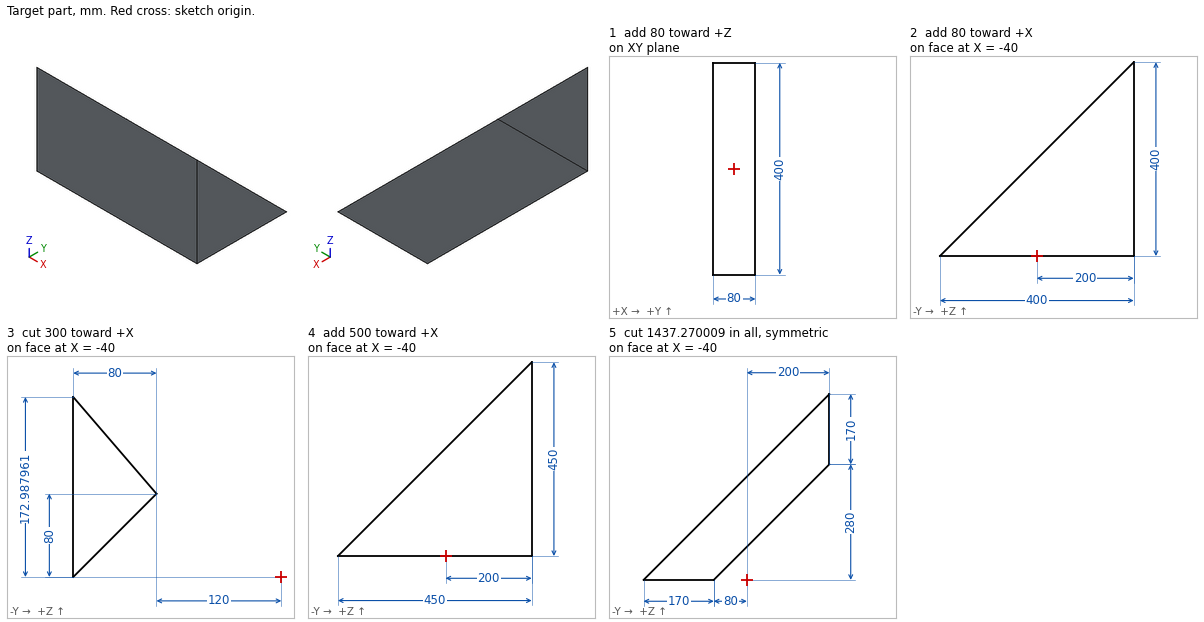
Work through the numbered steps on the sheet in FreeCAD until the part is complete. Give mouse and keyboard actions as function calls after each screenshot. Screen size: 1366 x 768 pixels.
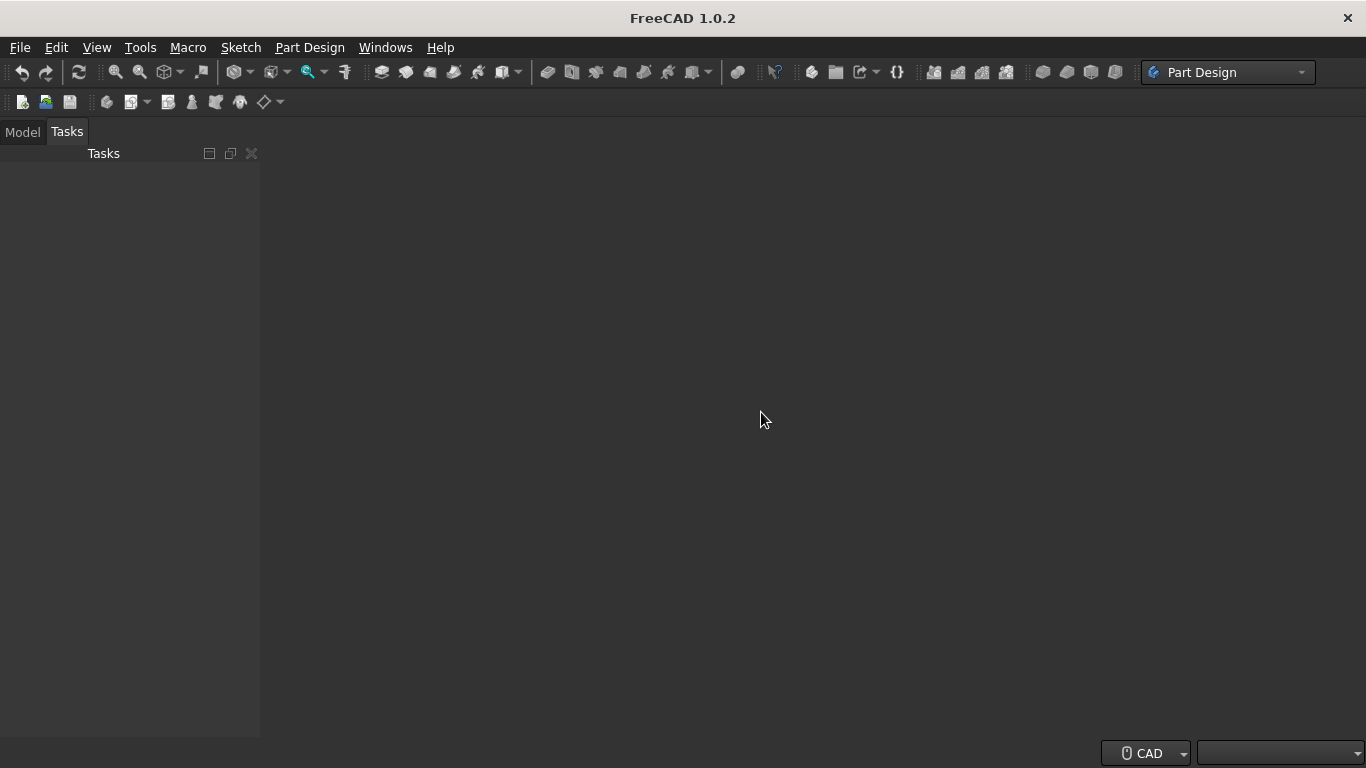
click(22, 102)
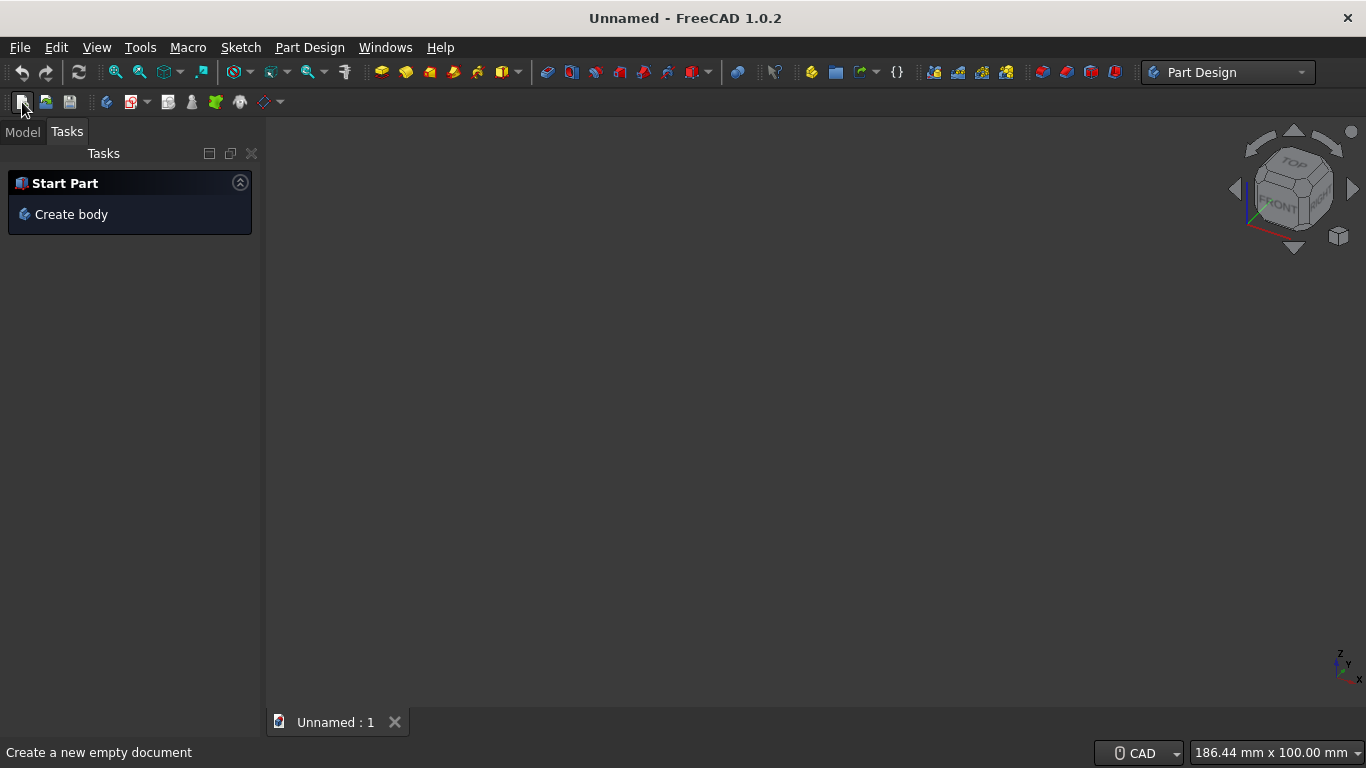
click(132, 102)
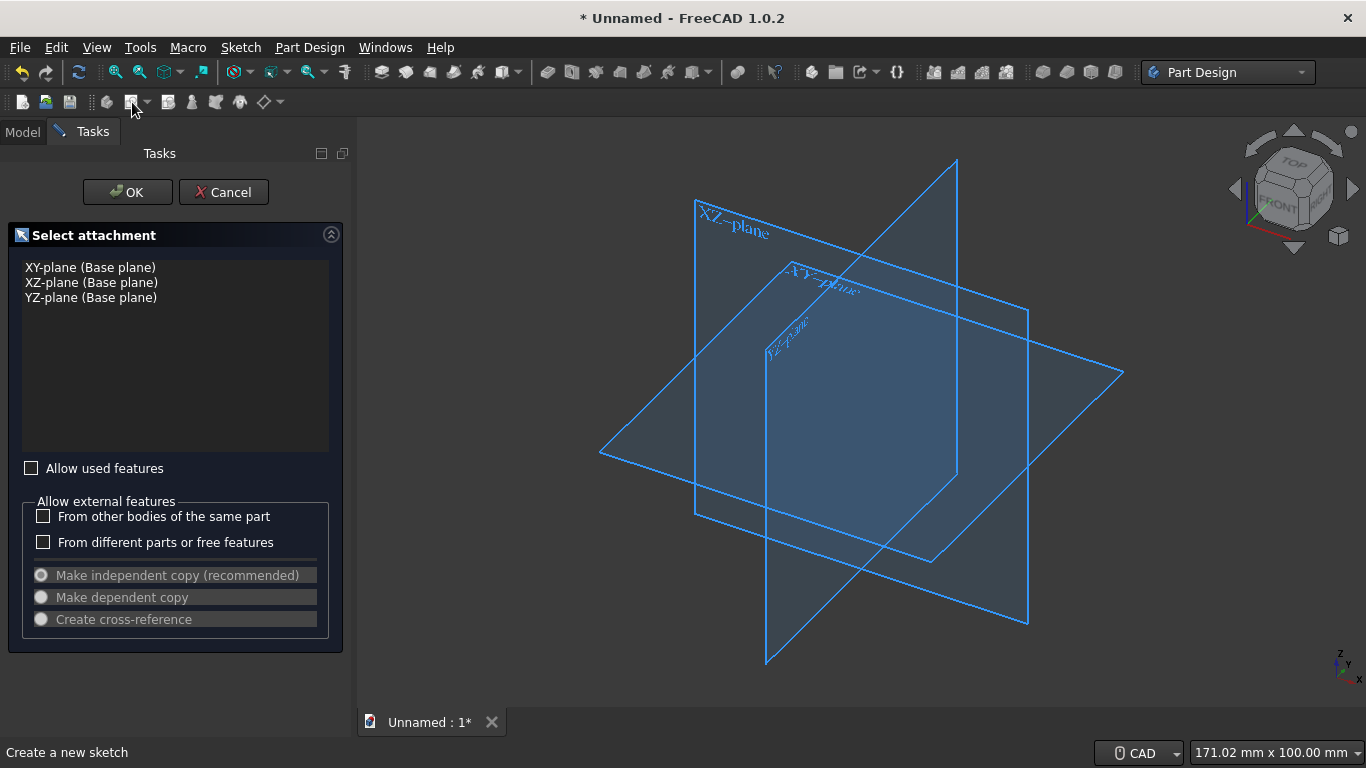
click(82, 268)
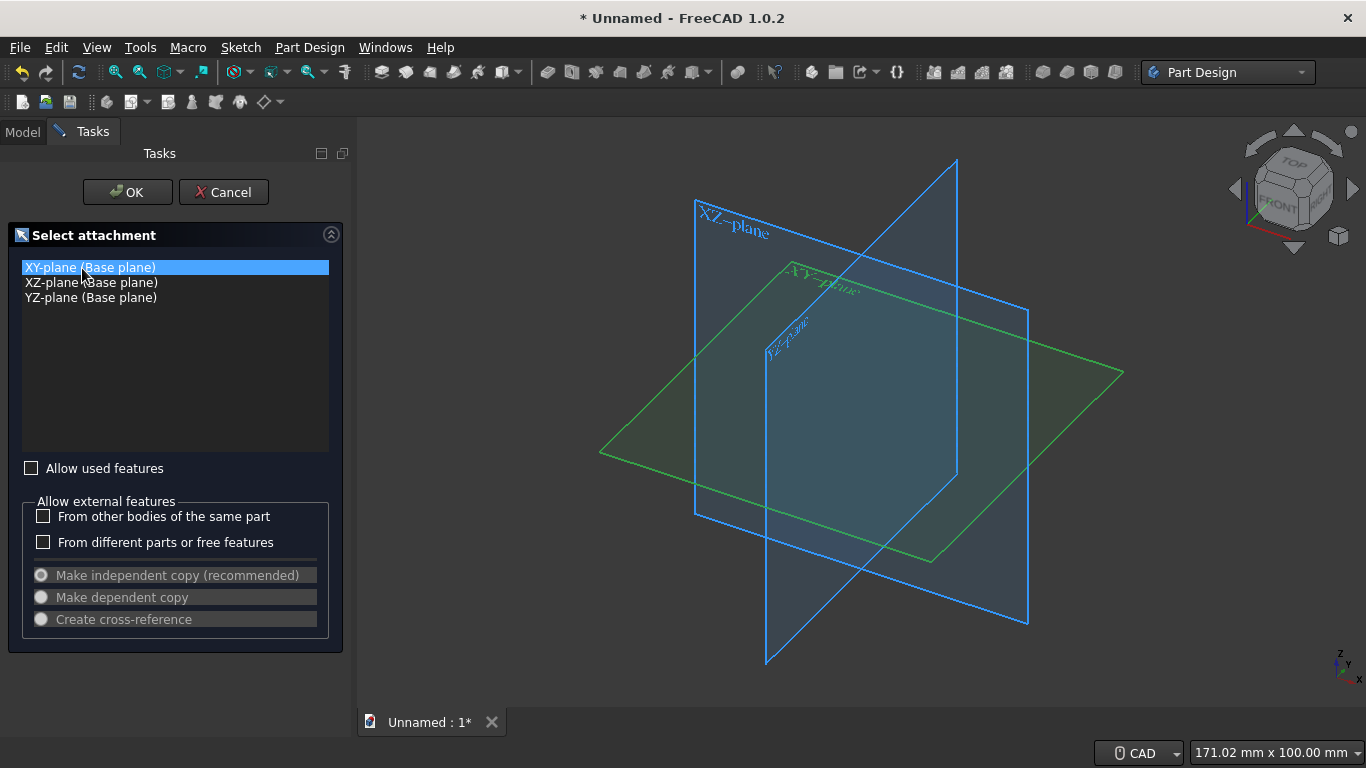
click(128, 192)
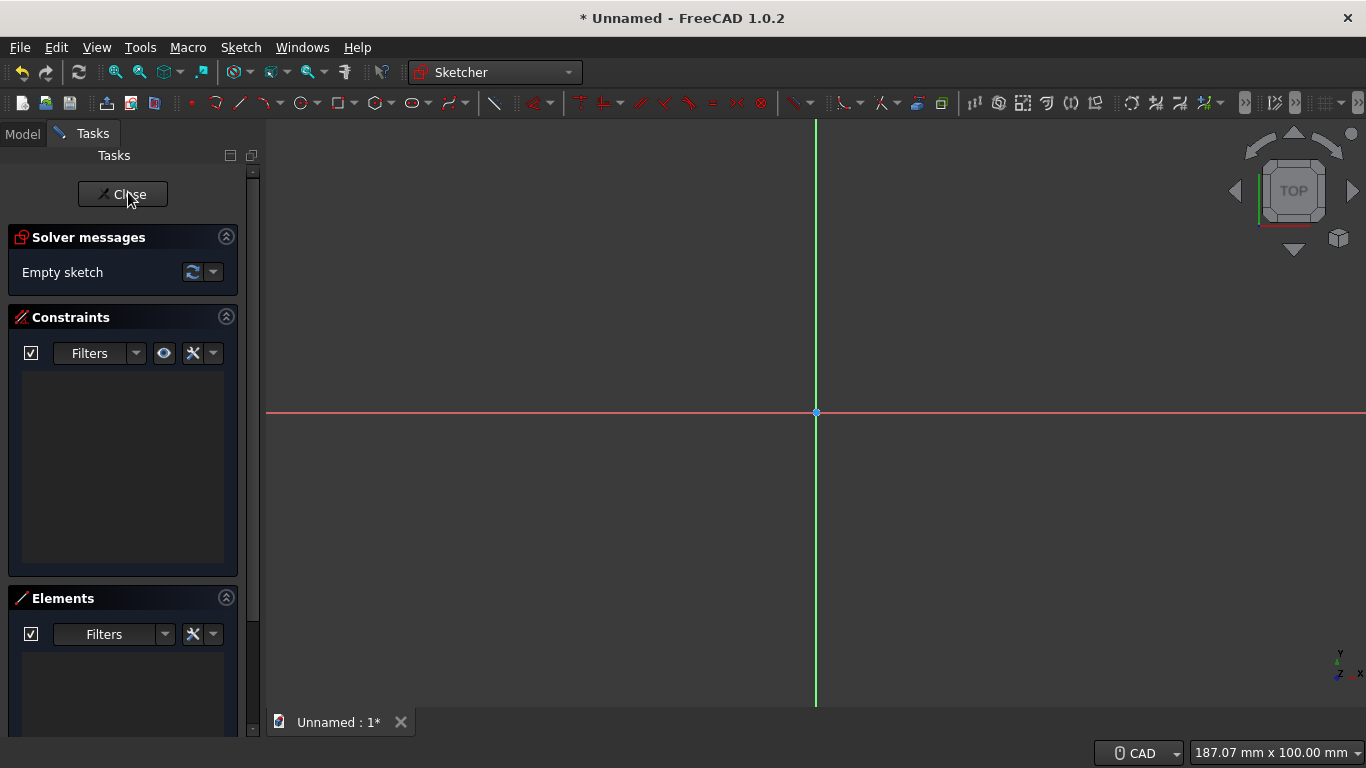
scroll(734, 413, down, 9)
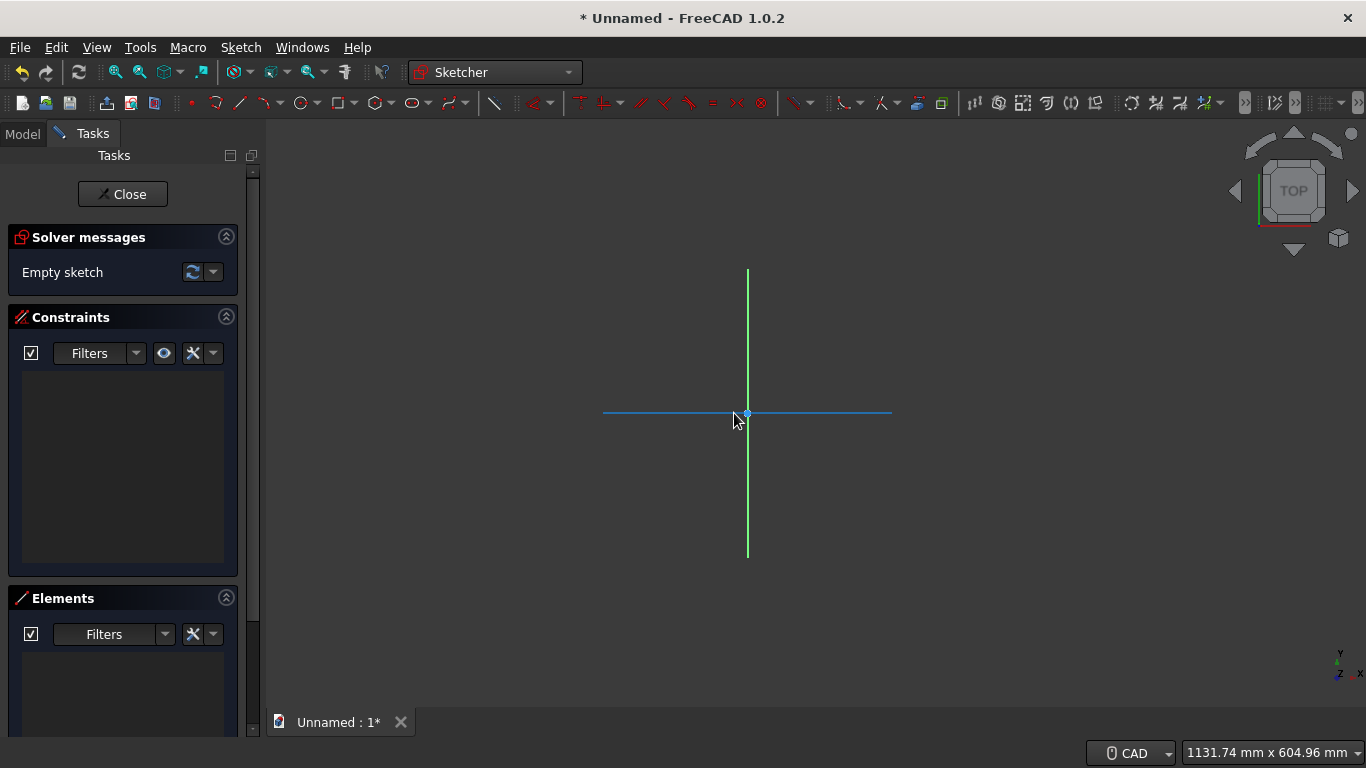
click(356, 104)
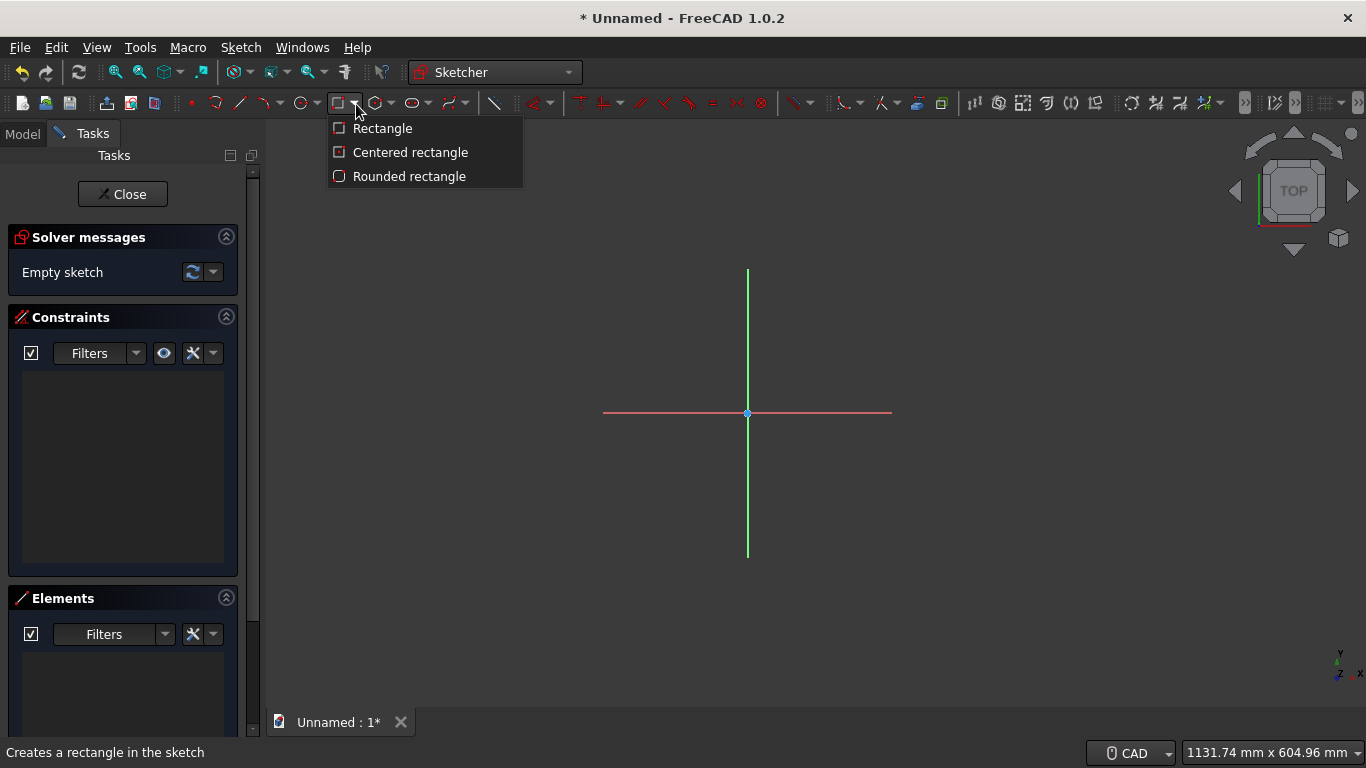
click(426, 152)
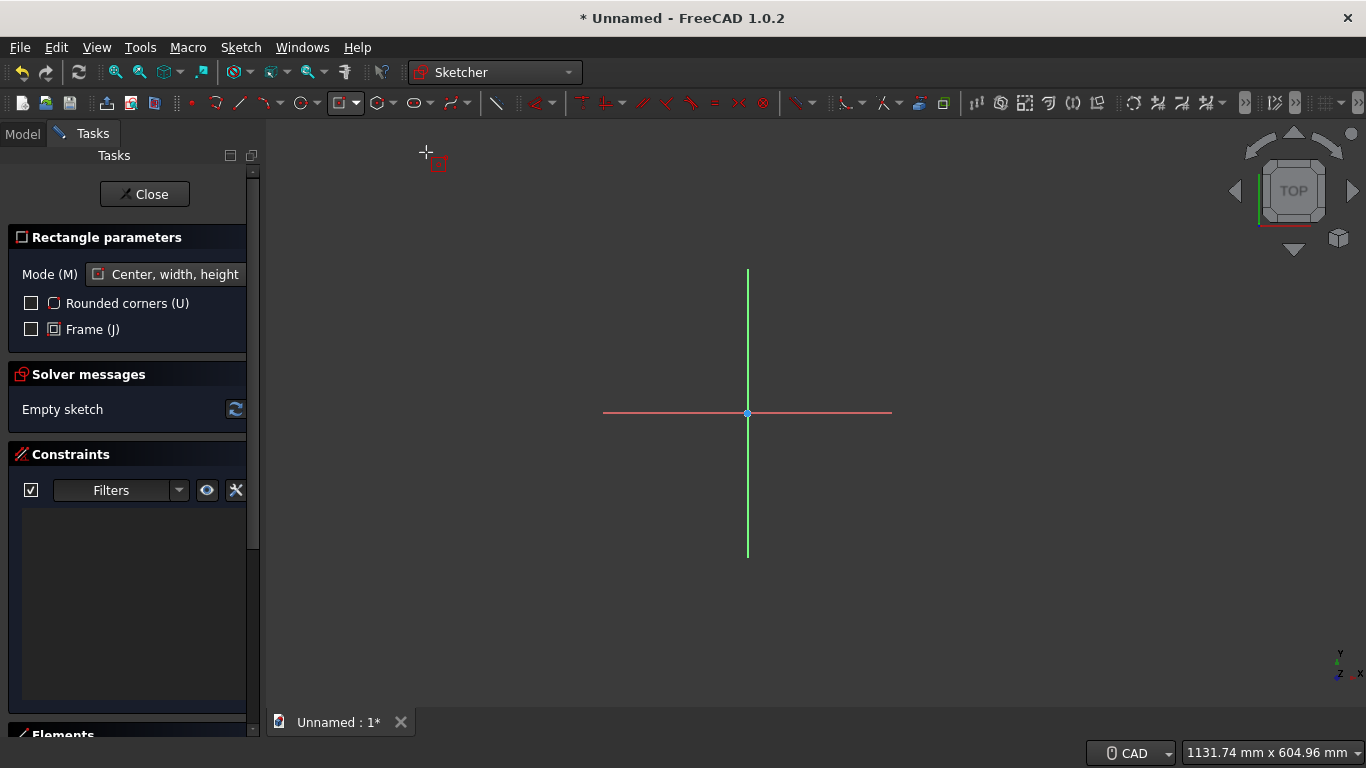
click(748, 413)
move(787, 219)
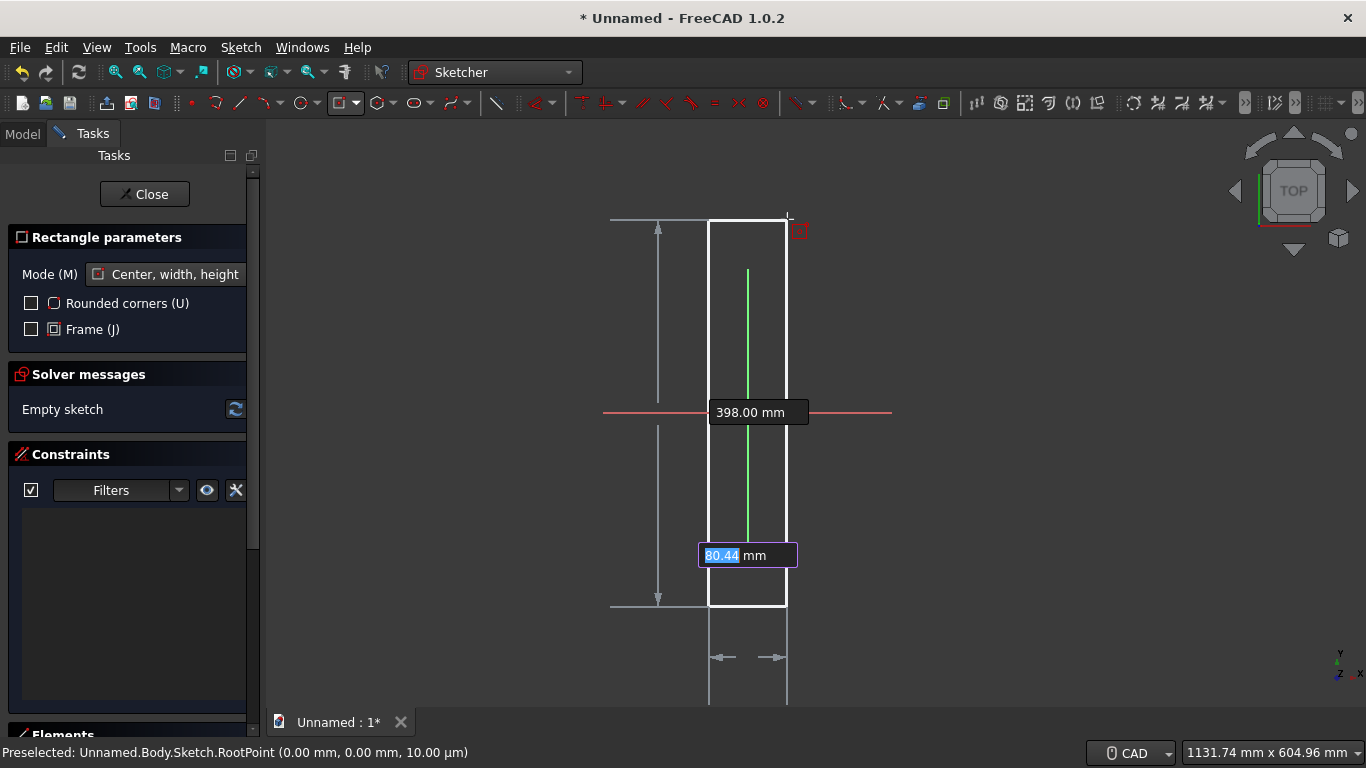
text(80)
key(Tab)
text(400)
key(Return)
key(Escape)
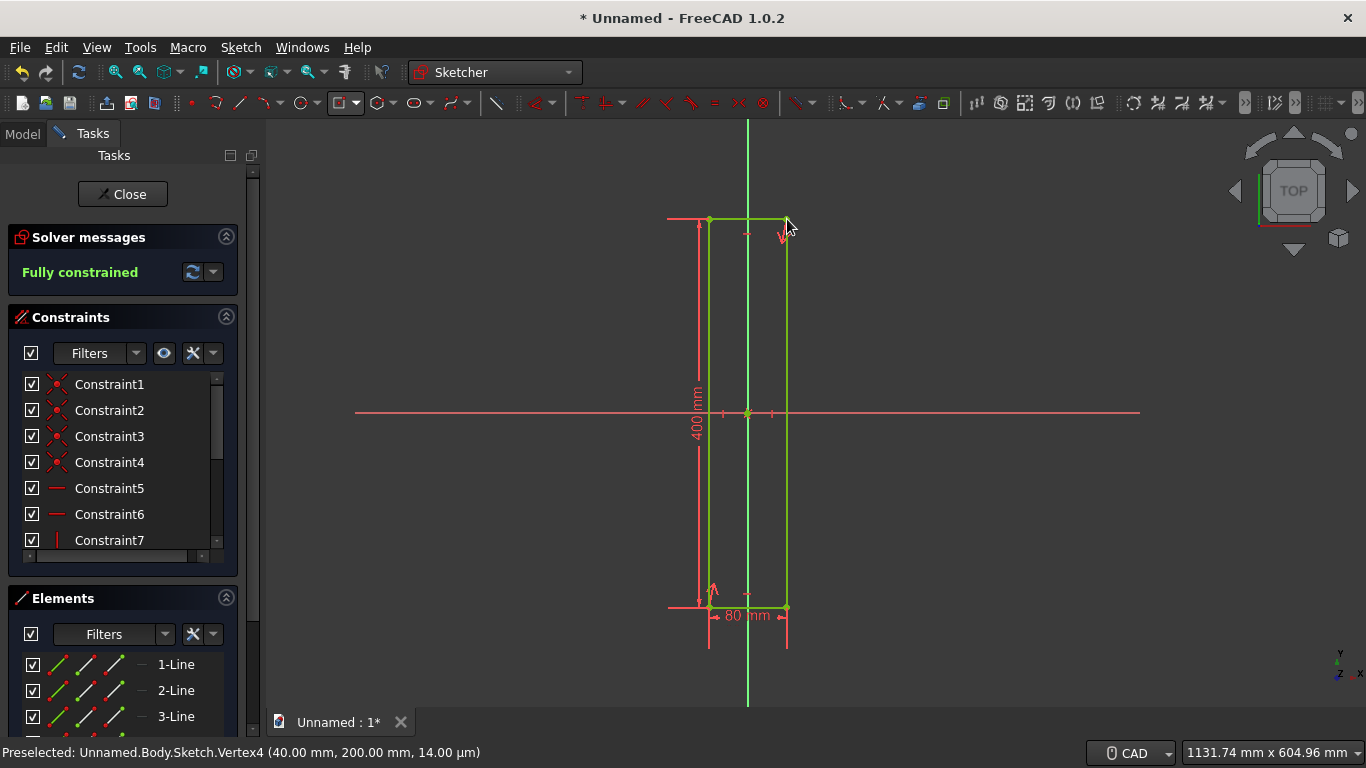
click(123, 194)